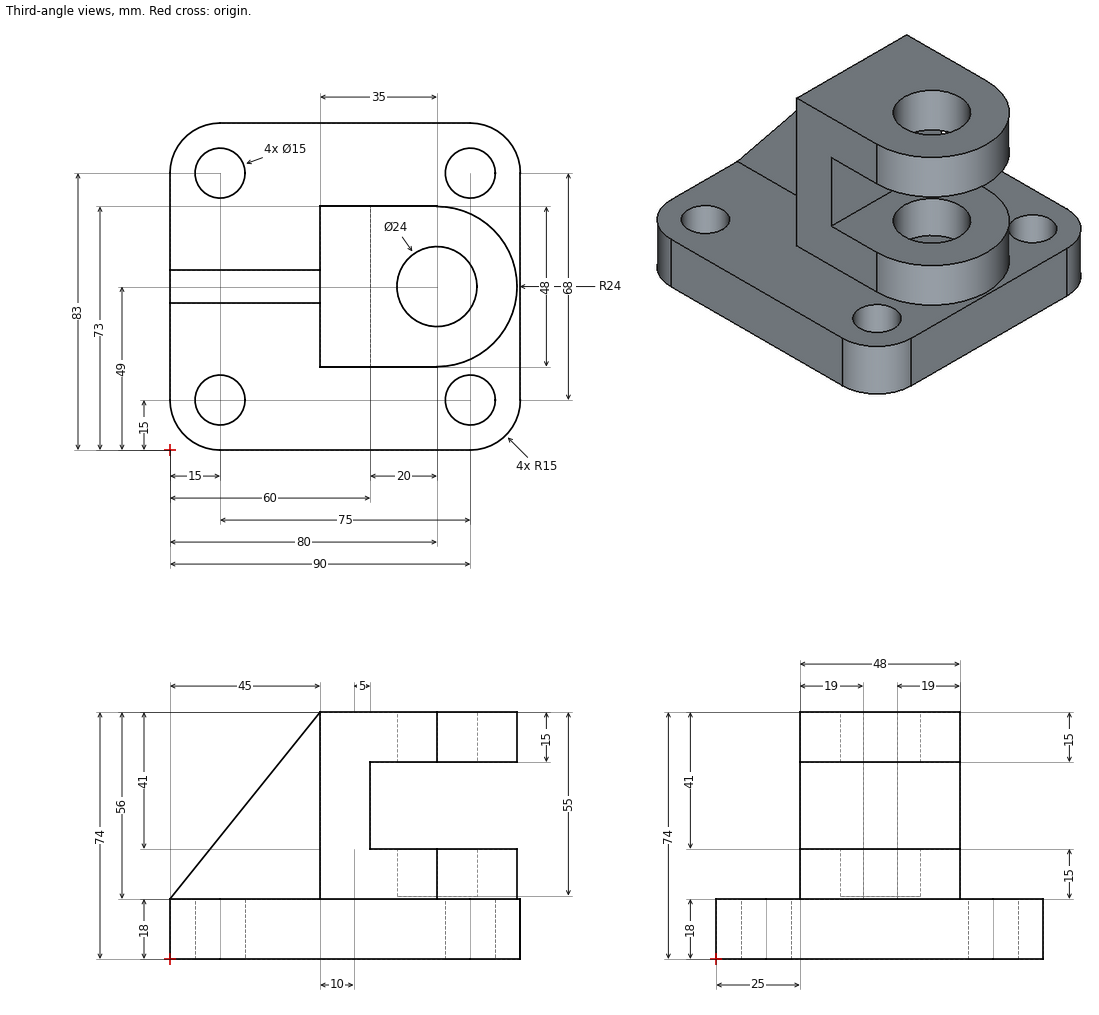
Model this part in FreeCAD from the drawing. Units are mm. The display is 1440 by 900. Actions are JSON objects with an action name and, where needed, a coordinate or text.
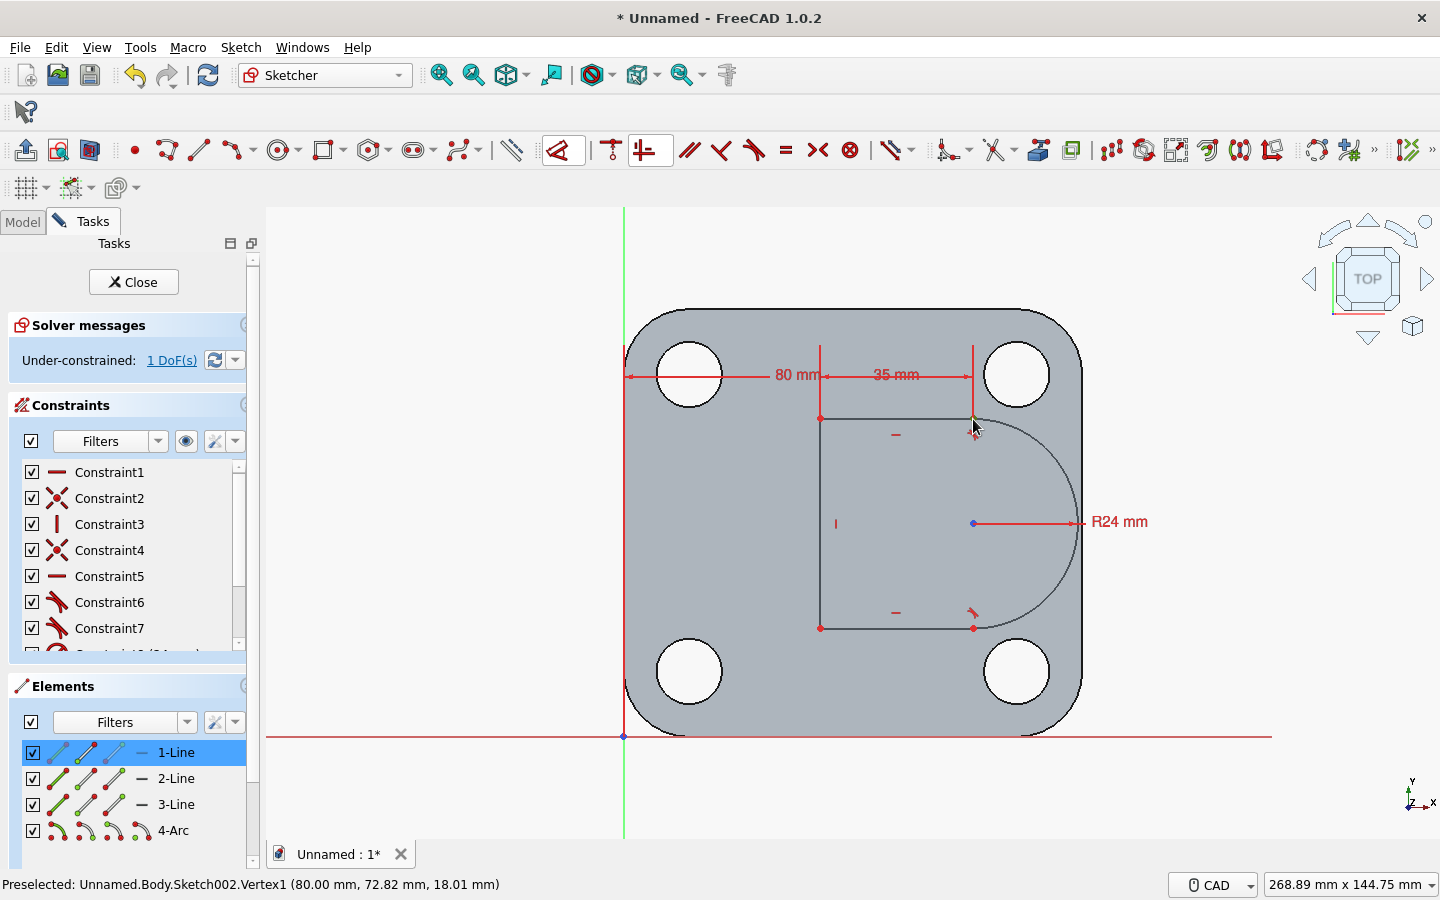
{"action": "key", "text": "i"}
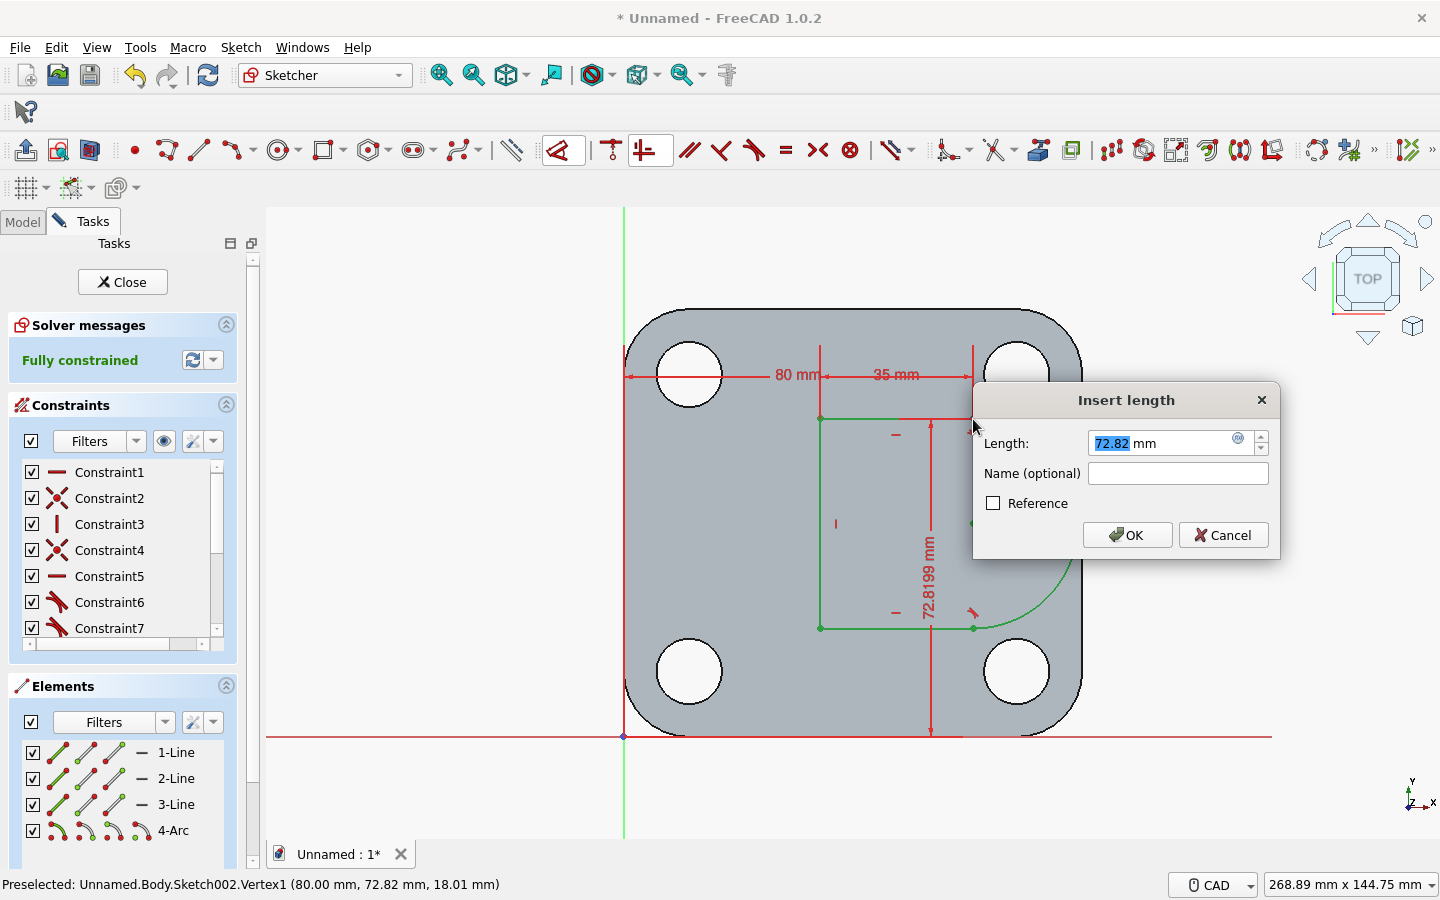
{"action": "type", "text": "73"}
{"action": "key", "text": "Return"}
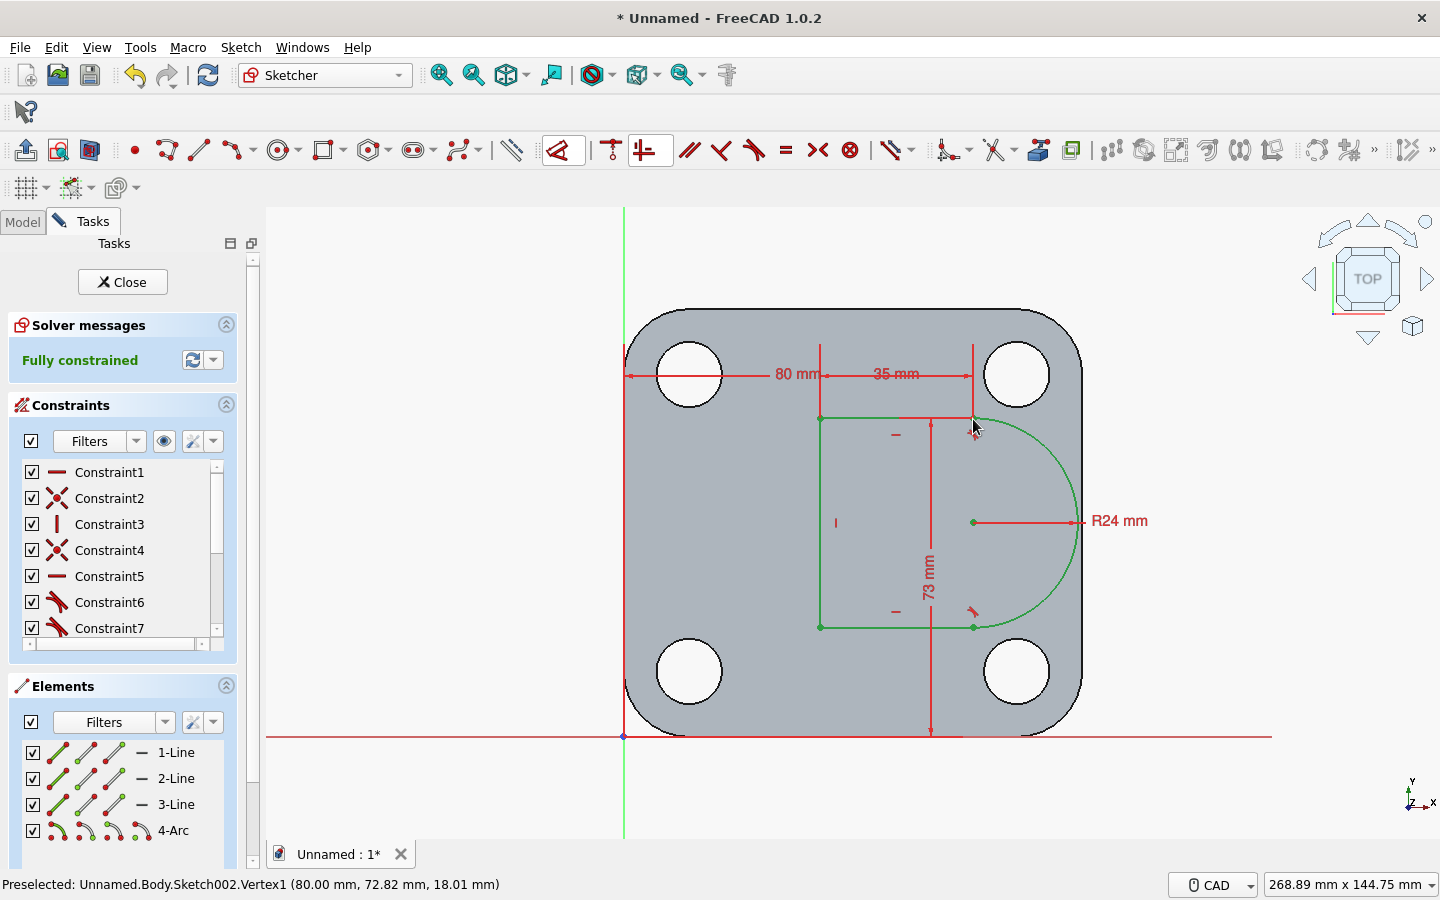
{"action": "left_click", "coordinate": [123, 282]}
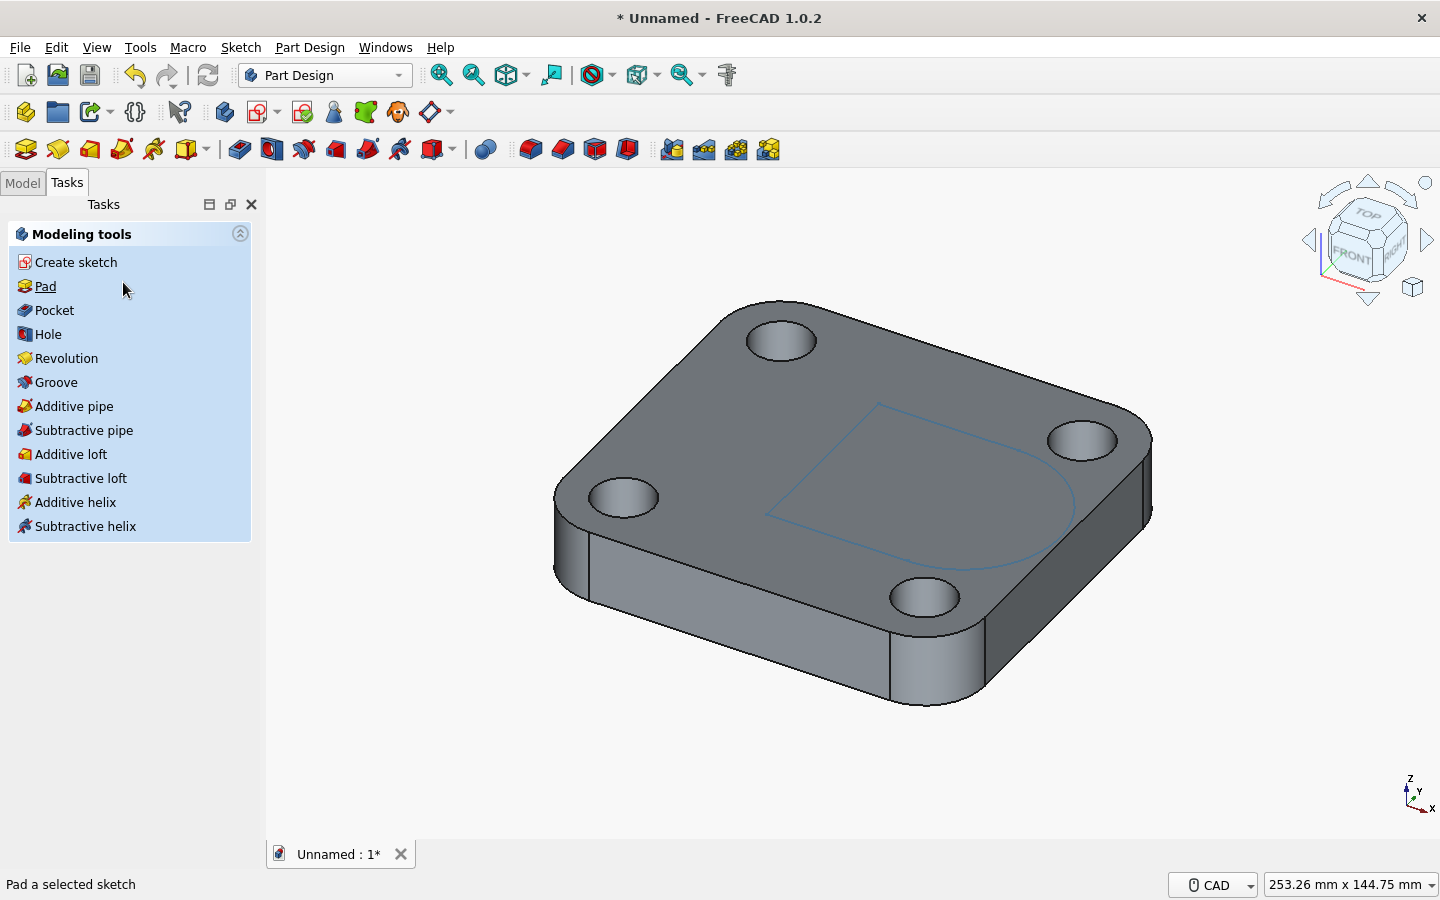
{"action": "left_click", "coordinate": [26, 150]}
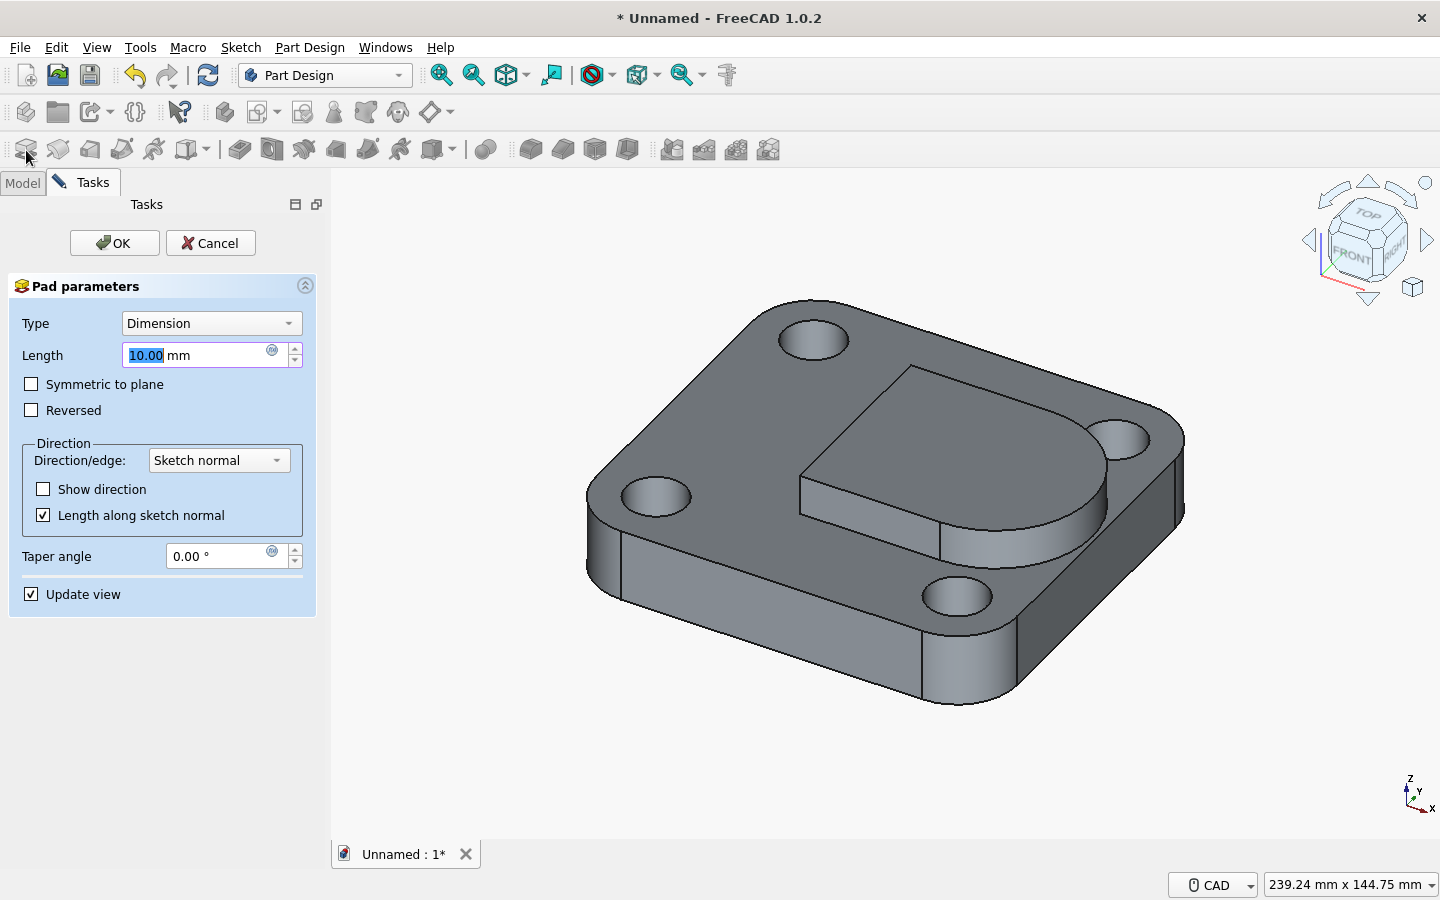
{"action": "type", "text": "15"}
{"action": "key", "text": "Tab"}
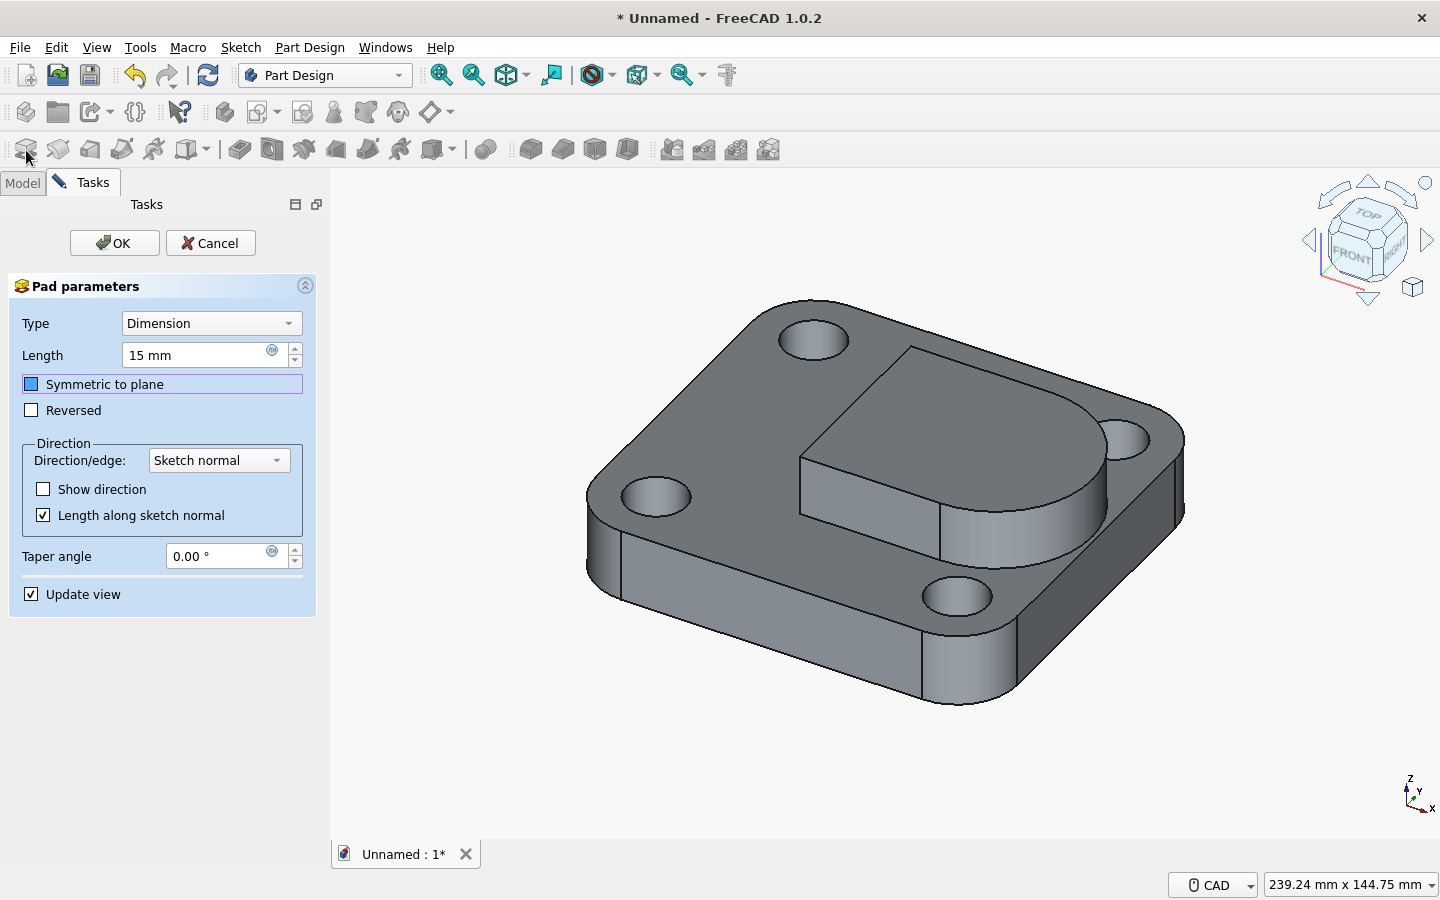
{"action": "left_click", "coordinate": [115, 243]}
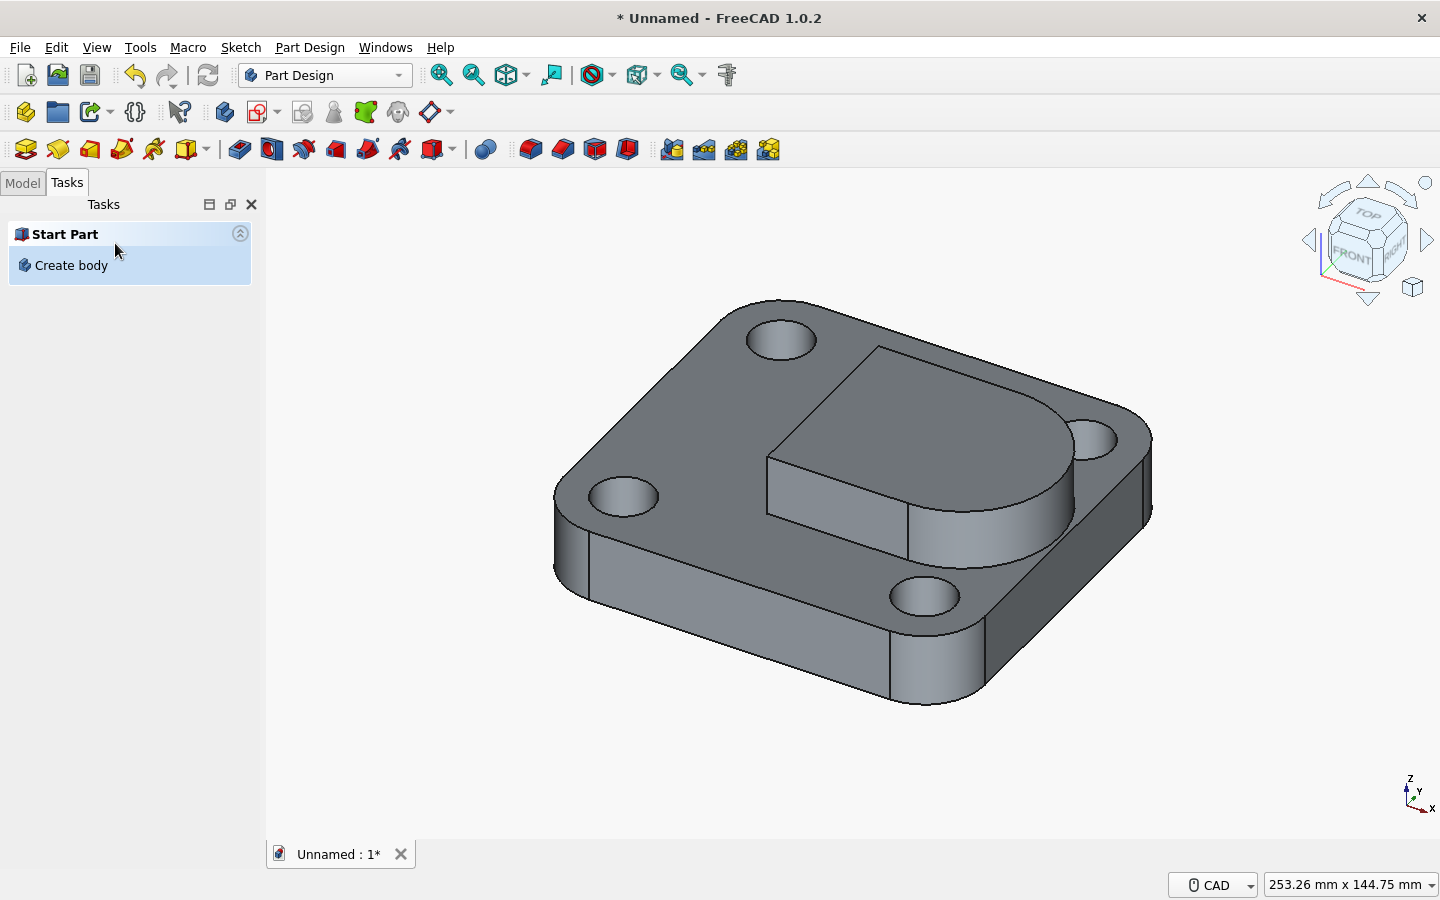
{"action": "left_click", "coordinate": [878, 521]}